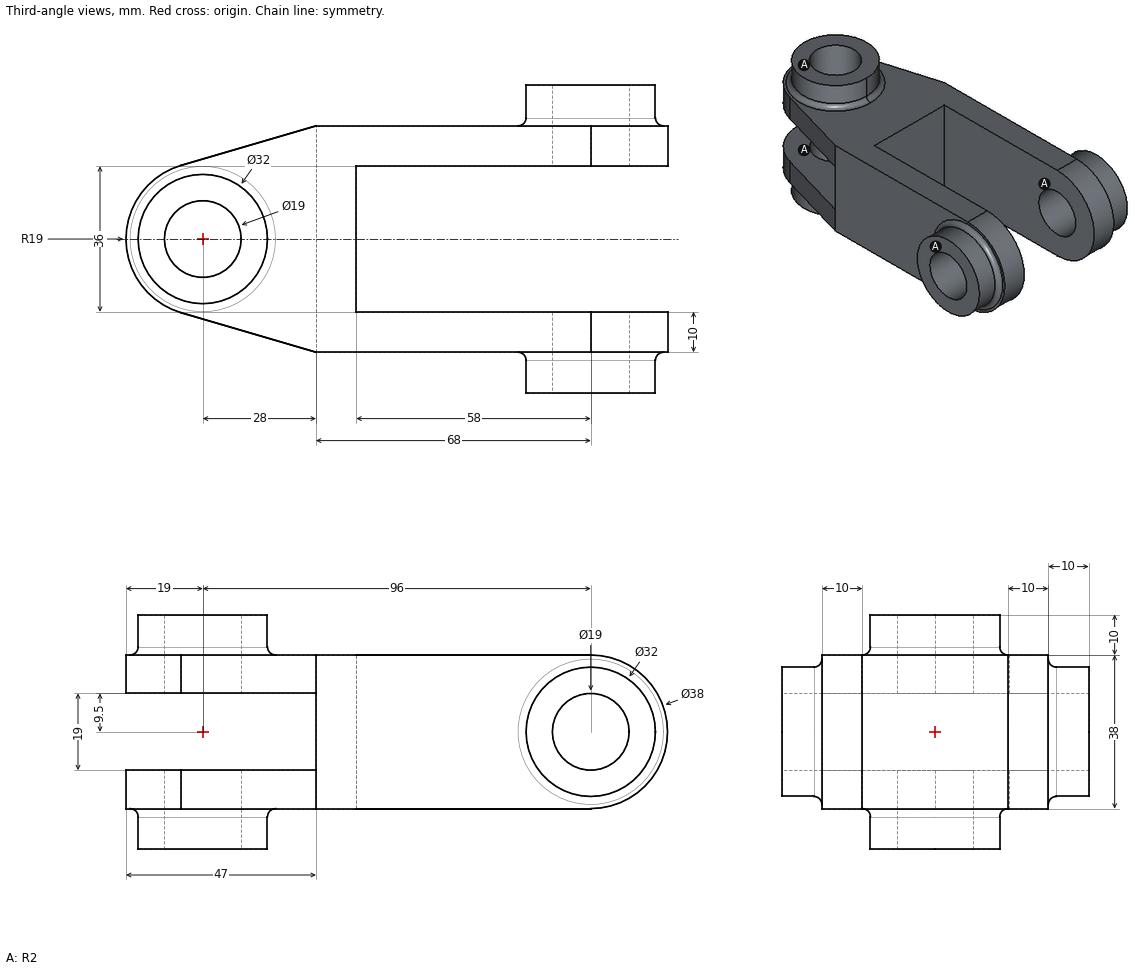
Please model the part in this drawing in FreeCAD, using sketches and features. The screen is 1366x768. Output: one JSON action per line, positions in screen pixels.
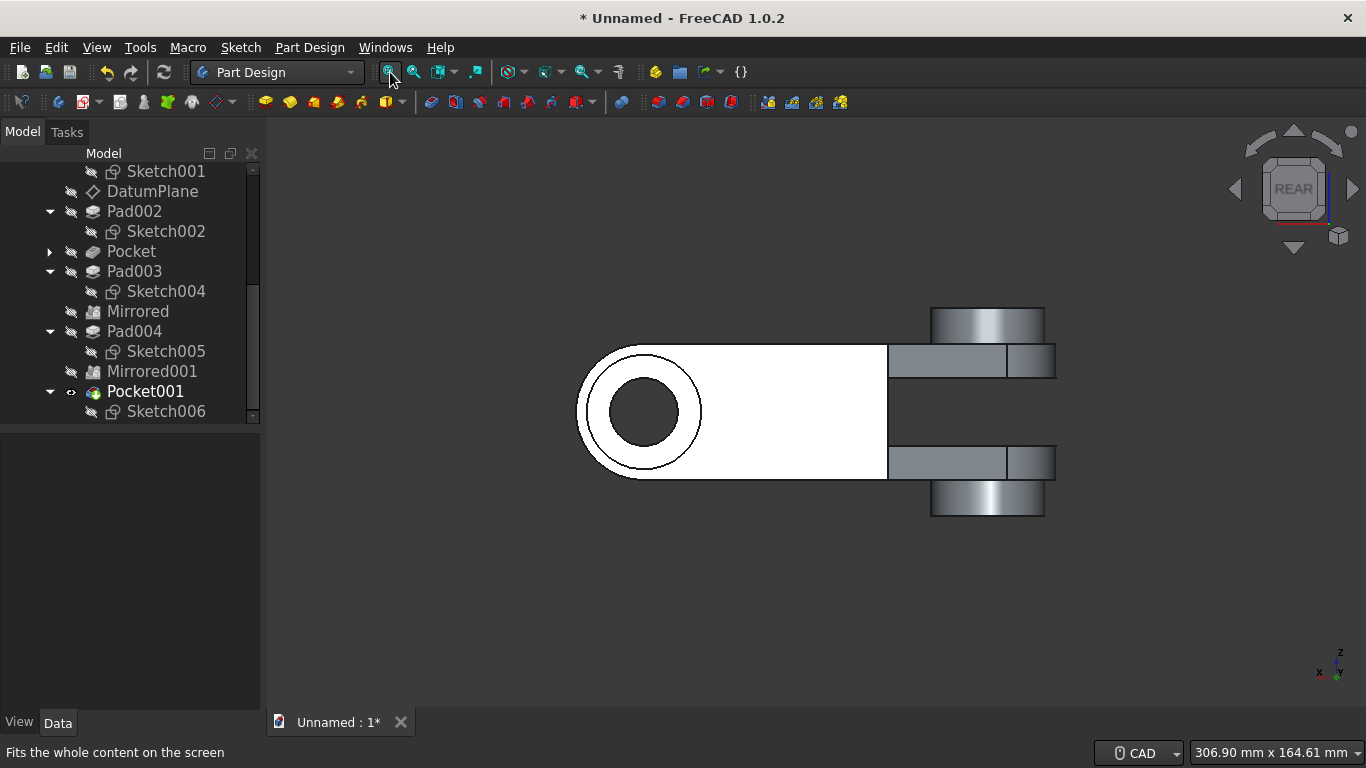
{"action": "left_click", "coordinate": [390, 72]}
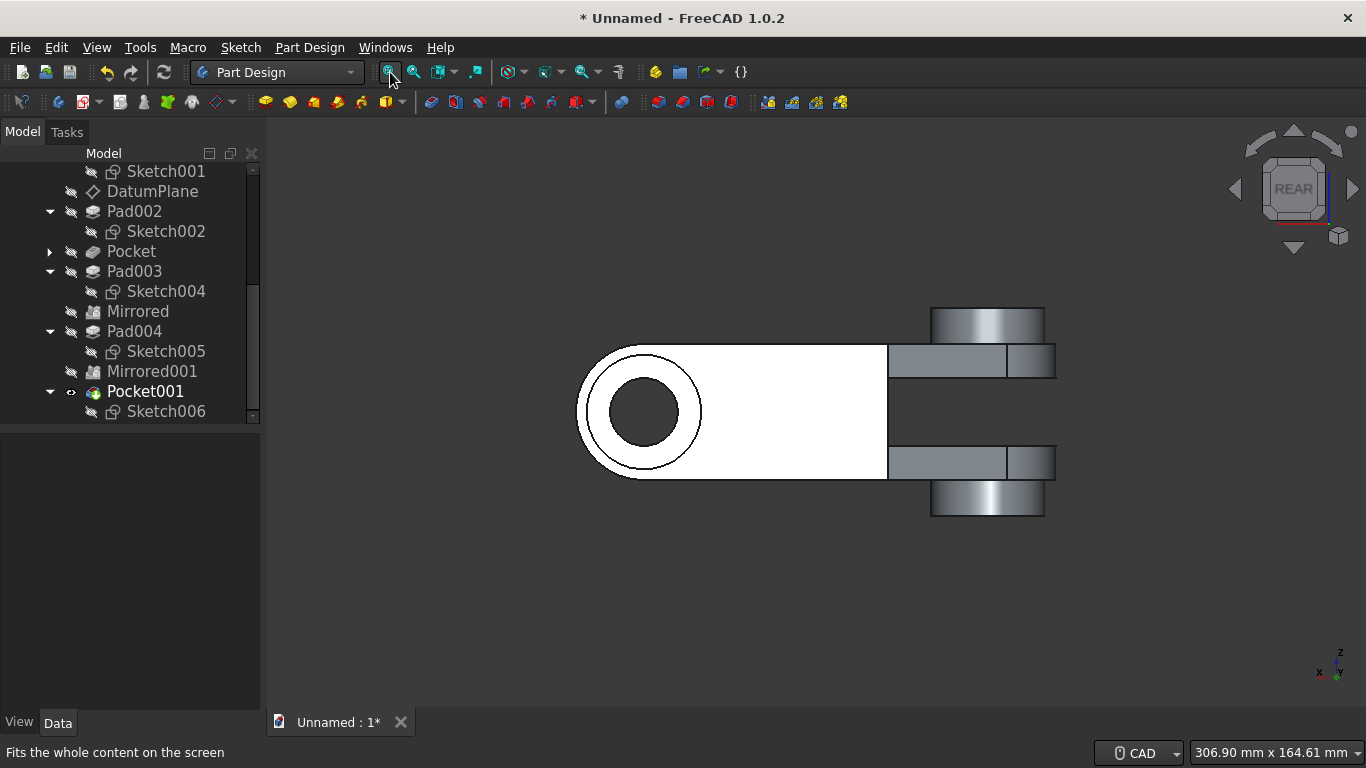
{"action": "key", "text": "6"}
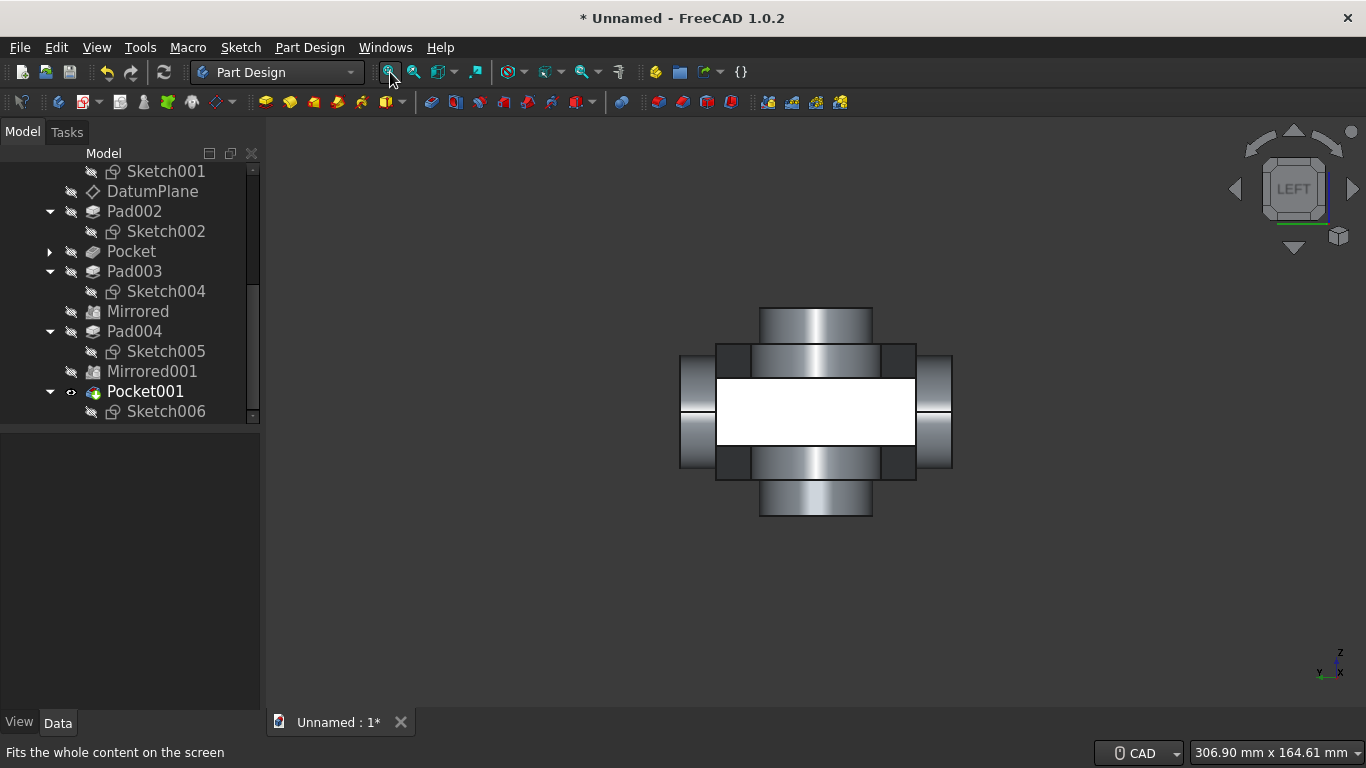
{"action": "left_click", "coordinate": [390, 72]}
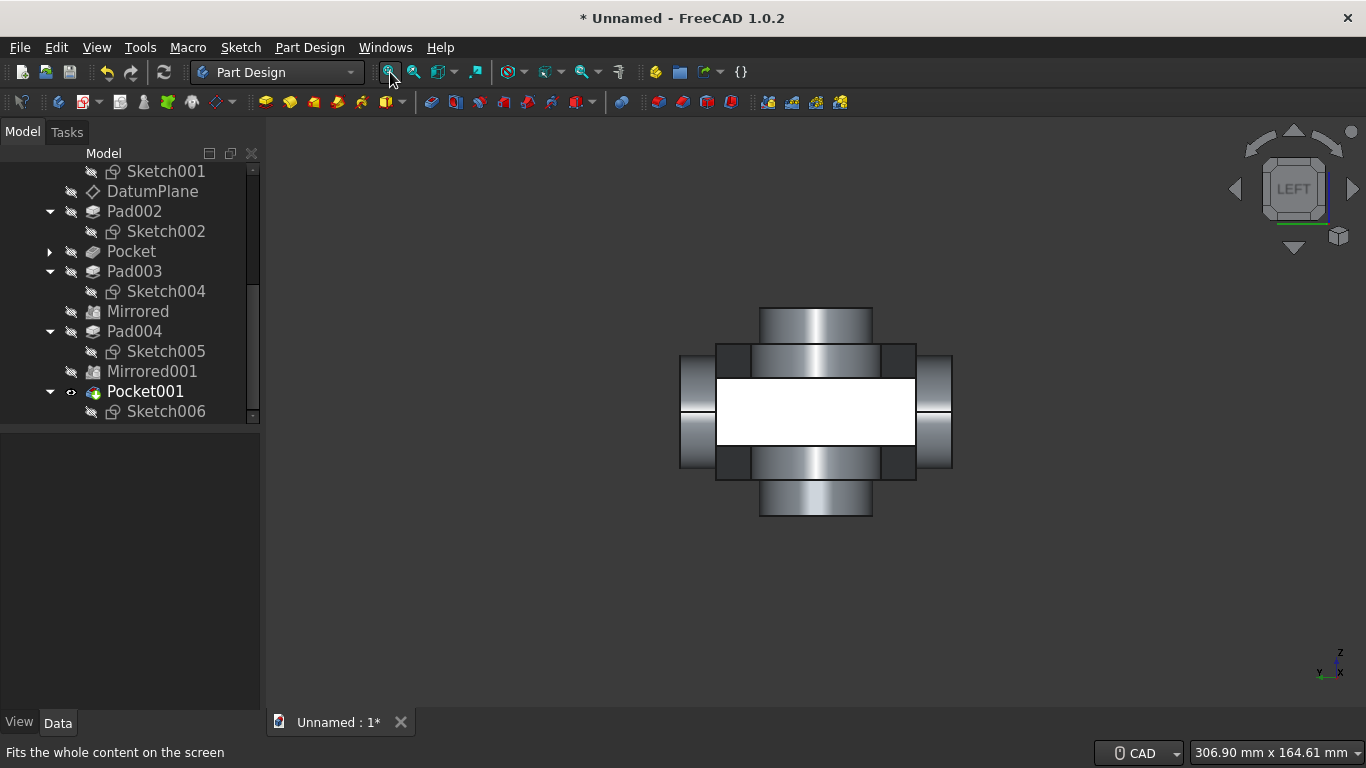
{"action": "key", "text": "v 3"}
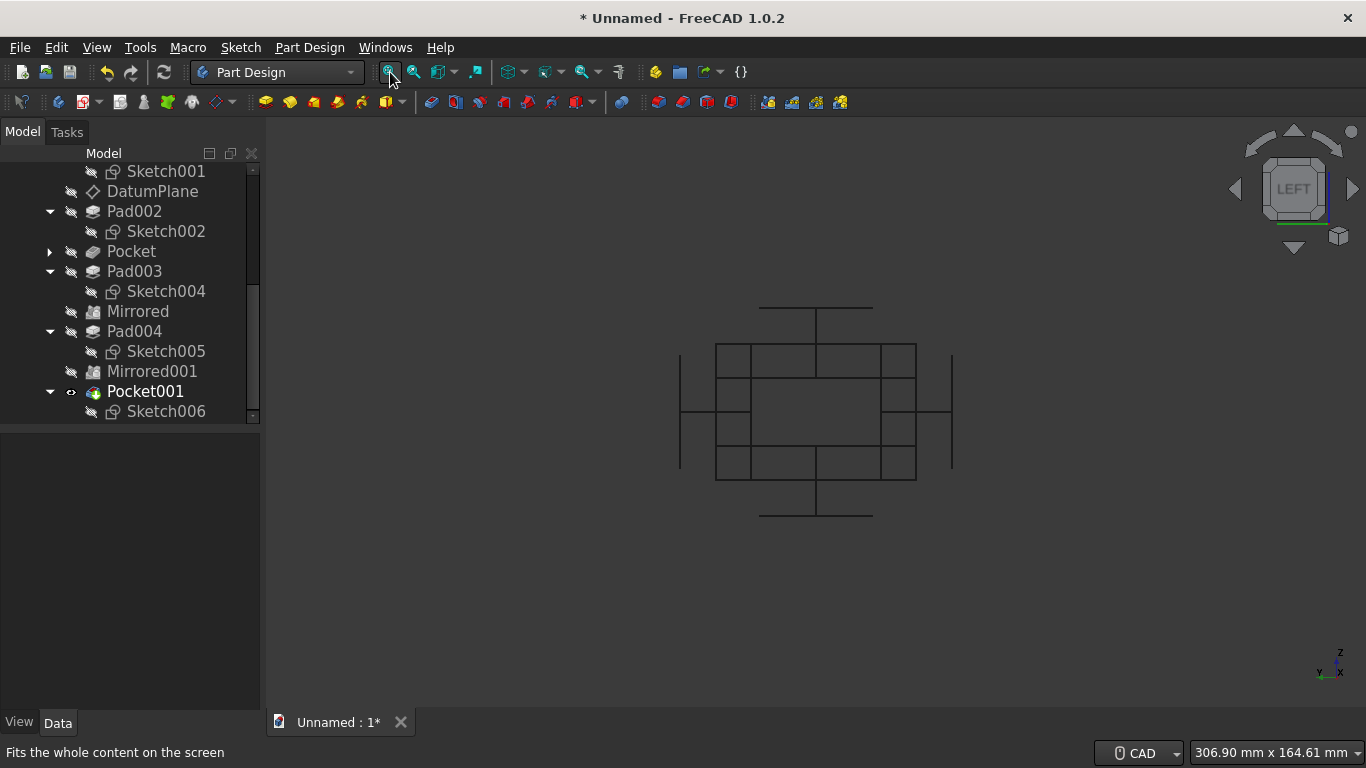
{"action": "key", "text": "0"}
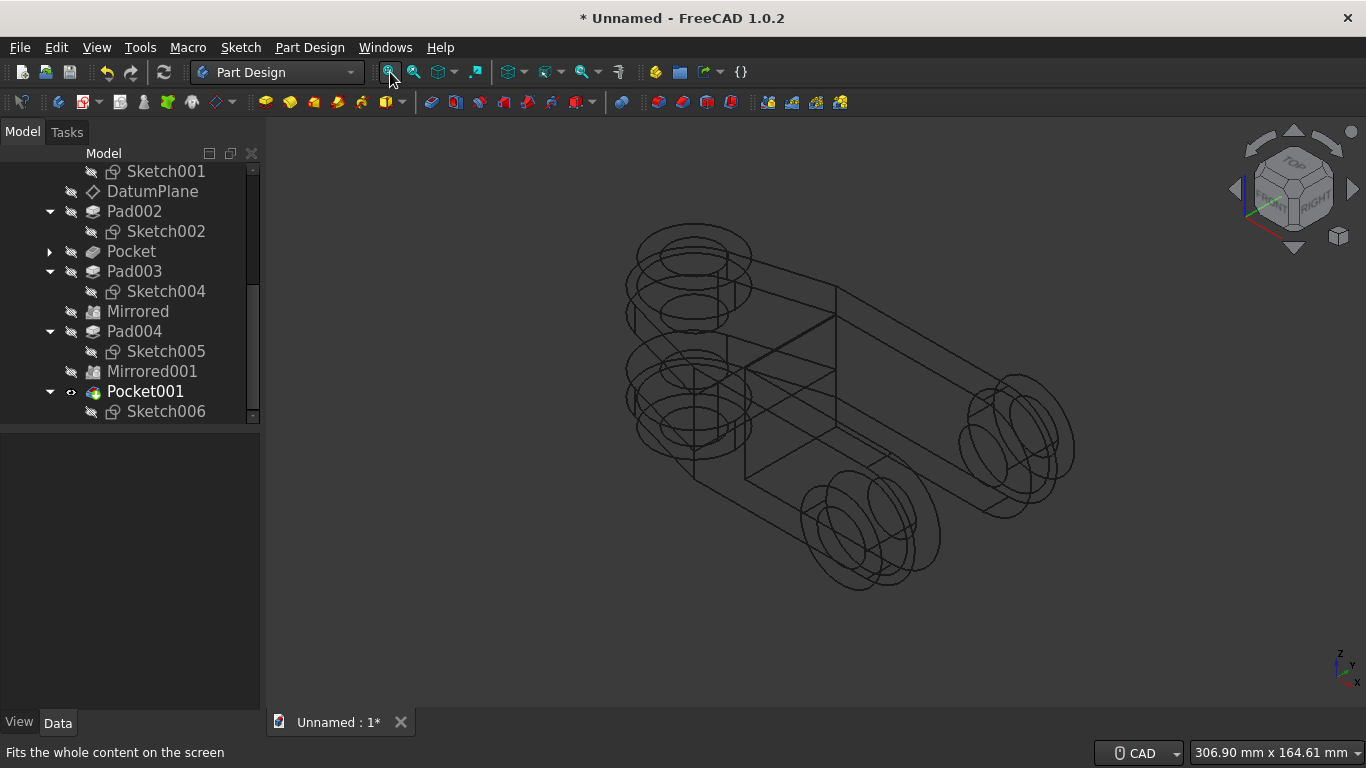
{"action": "left_click", "coordinate": [907, 546]}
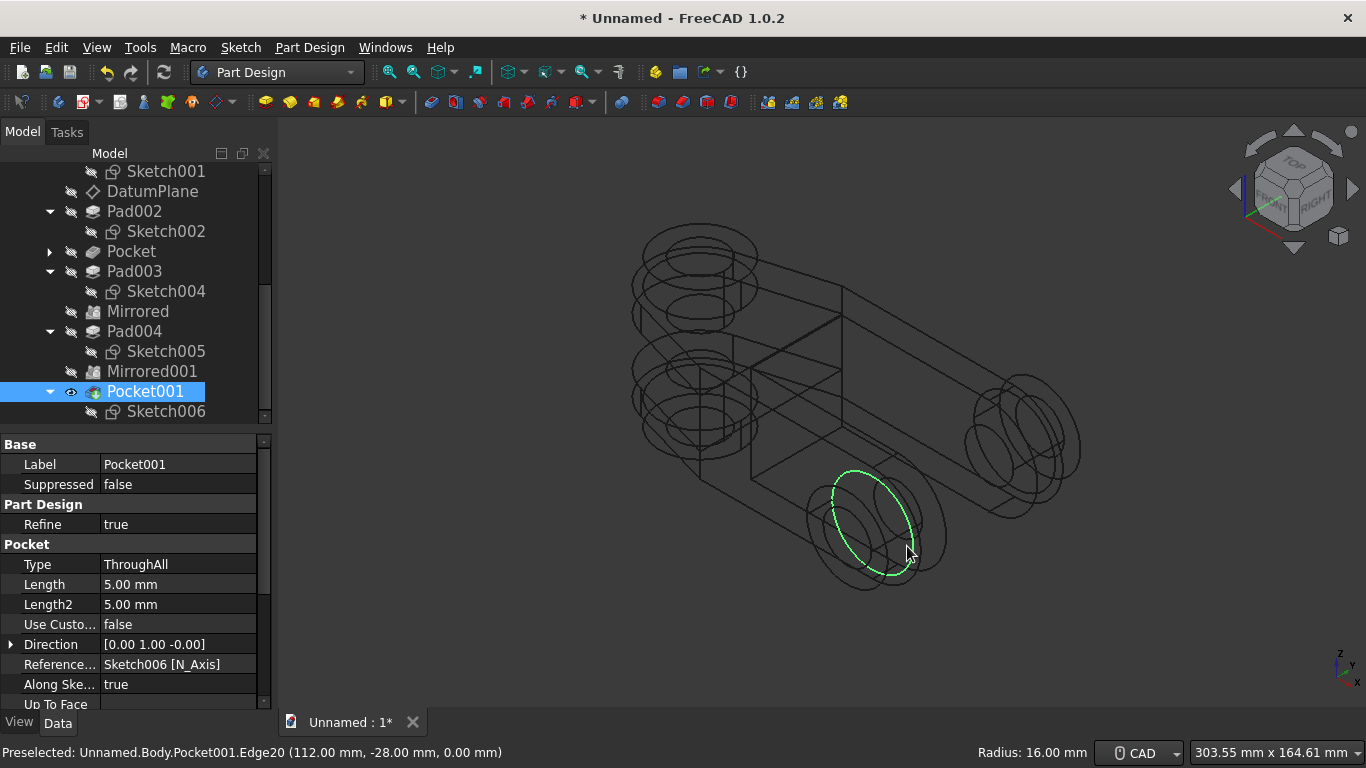
{"action": "left_click", "coordinate": [660, 262], "text": "ctrl"}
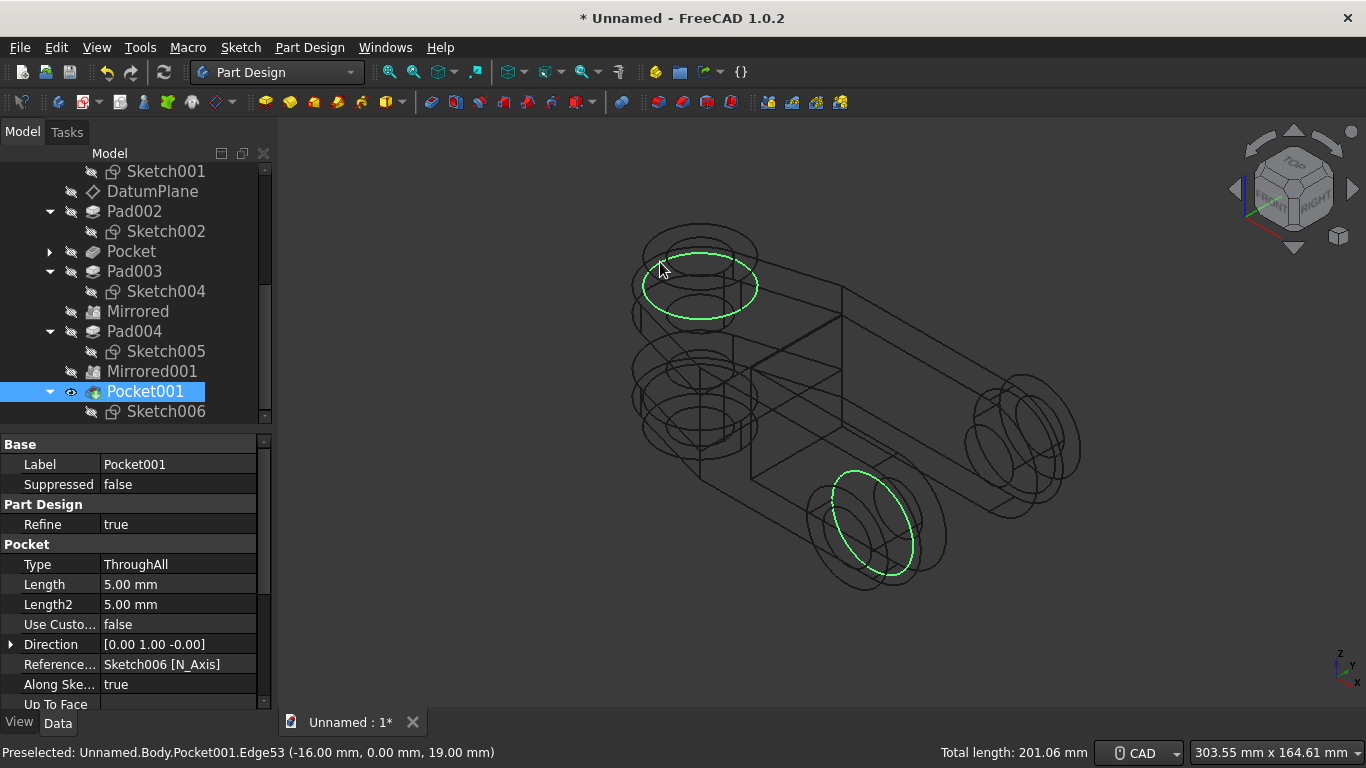
{"action": "left_click", "coordinate": [660, 373], "text": "ctrl"}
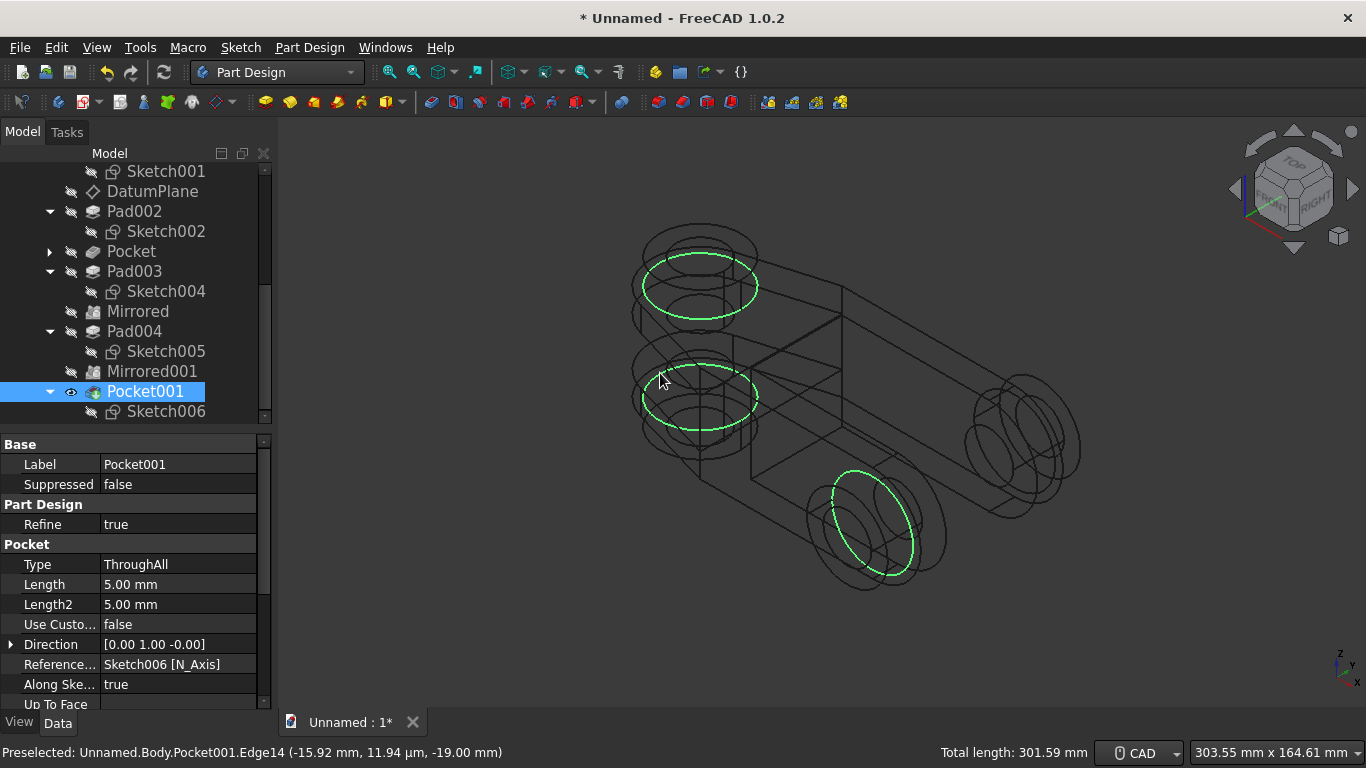
{"action": "left_click", "coordinate": [1055, 464], "text": "ctrl"}